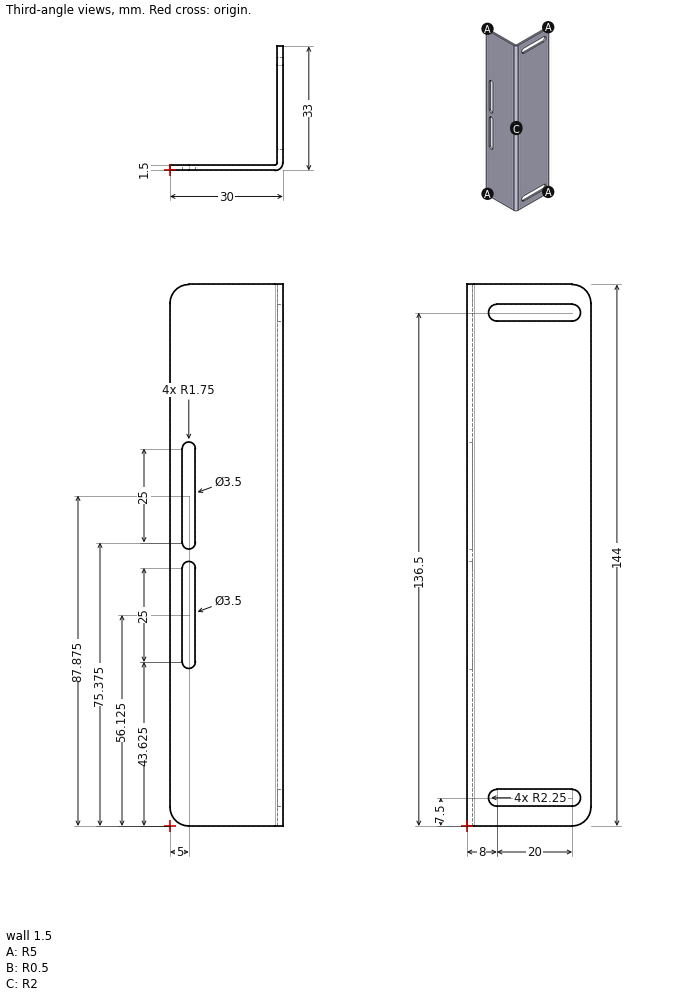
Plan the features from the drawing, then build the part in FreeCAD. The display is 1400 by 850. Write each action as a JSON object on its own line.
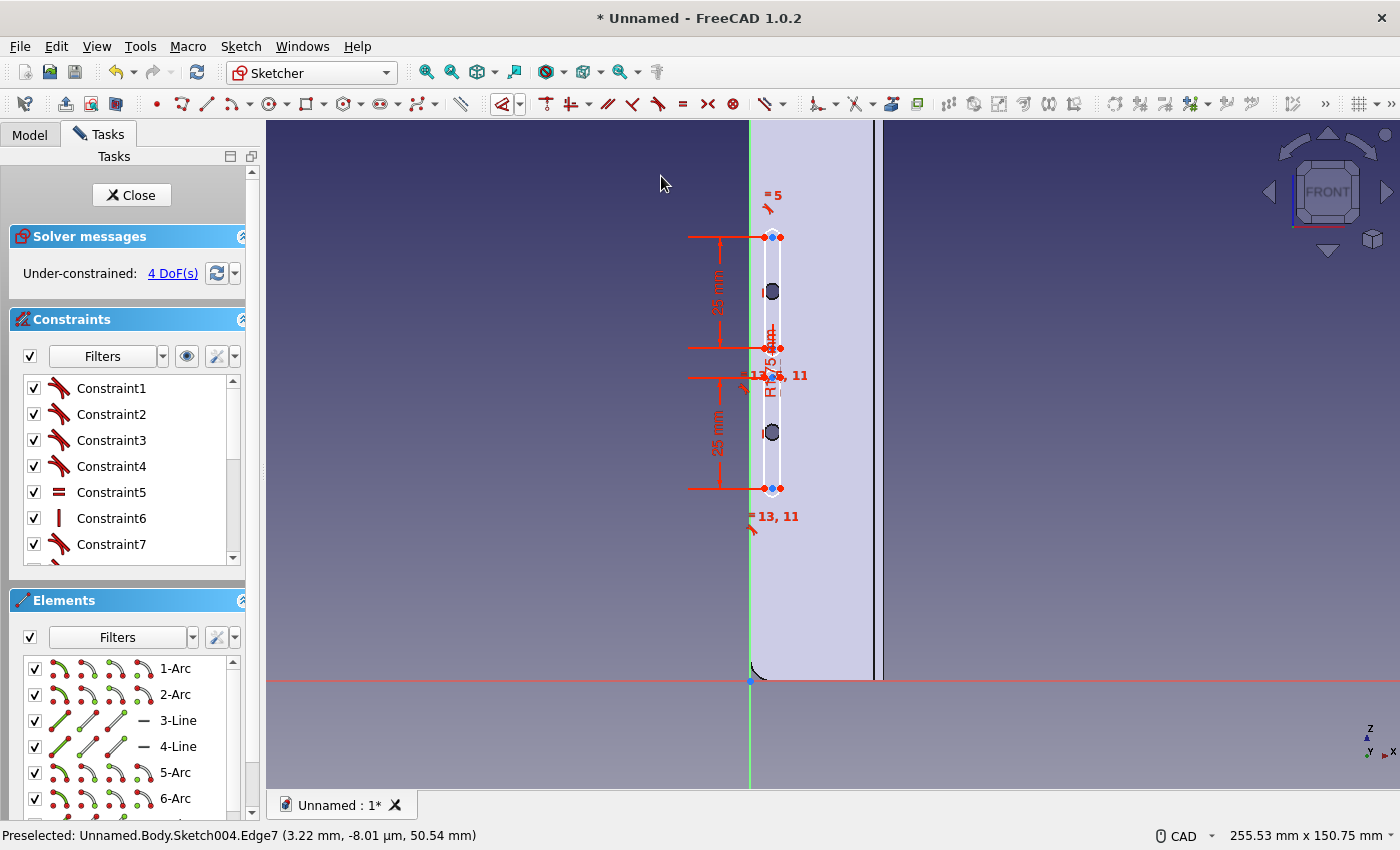
{"action": "scroll", "coordinate": [773, 348], "scroll_direction": "up", "scroll_amount": 3}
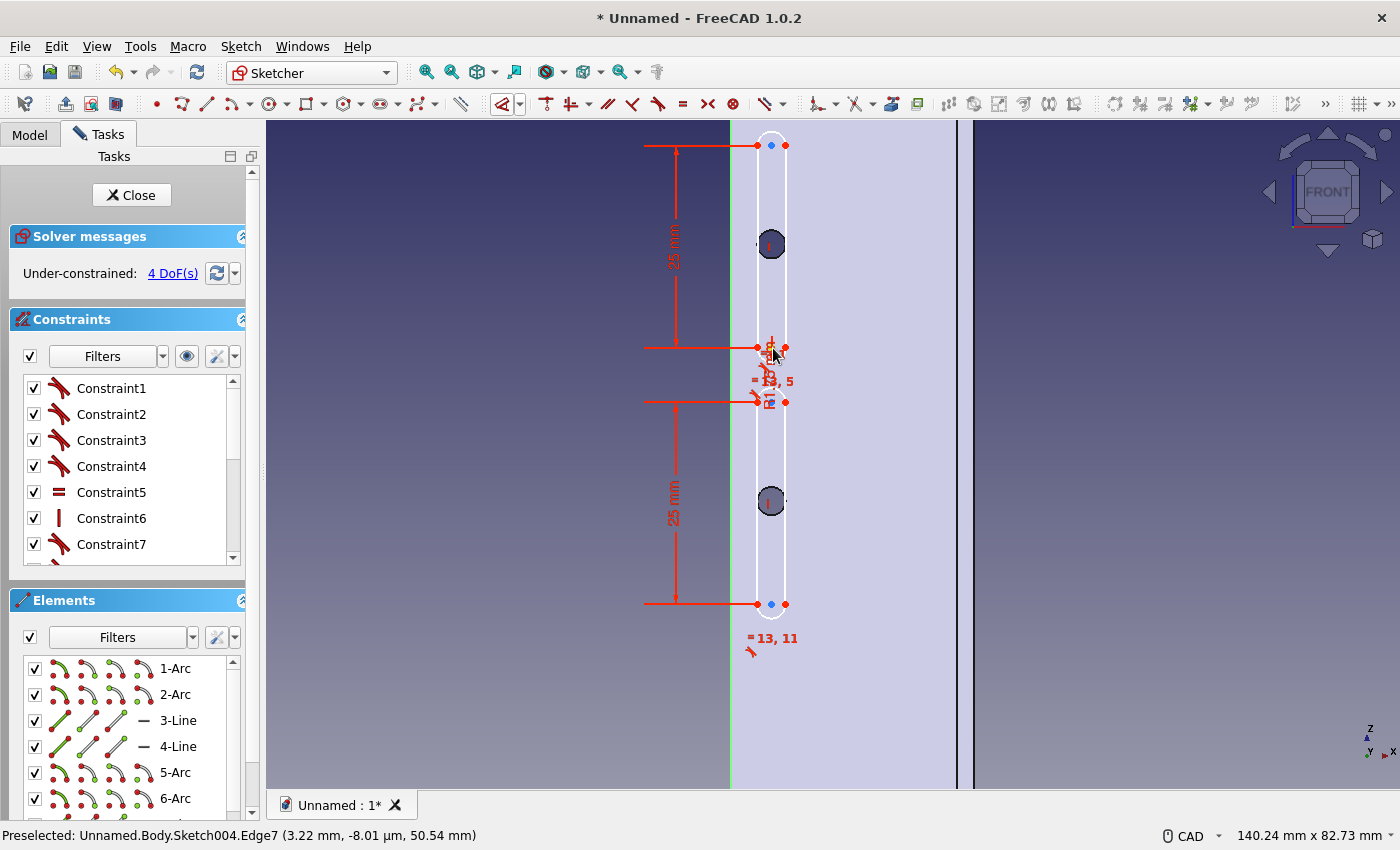
{"action": "scroll", "coordinate": [772, 348], "scroll_direction": "up", "scroll_amount": 4}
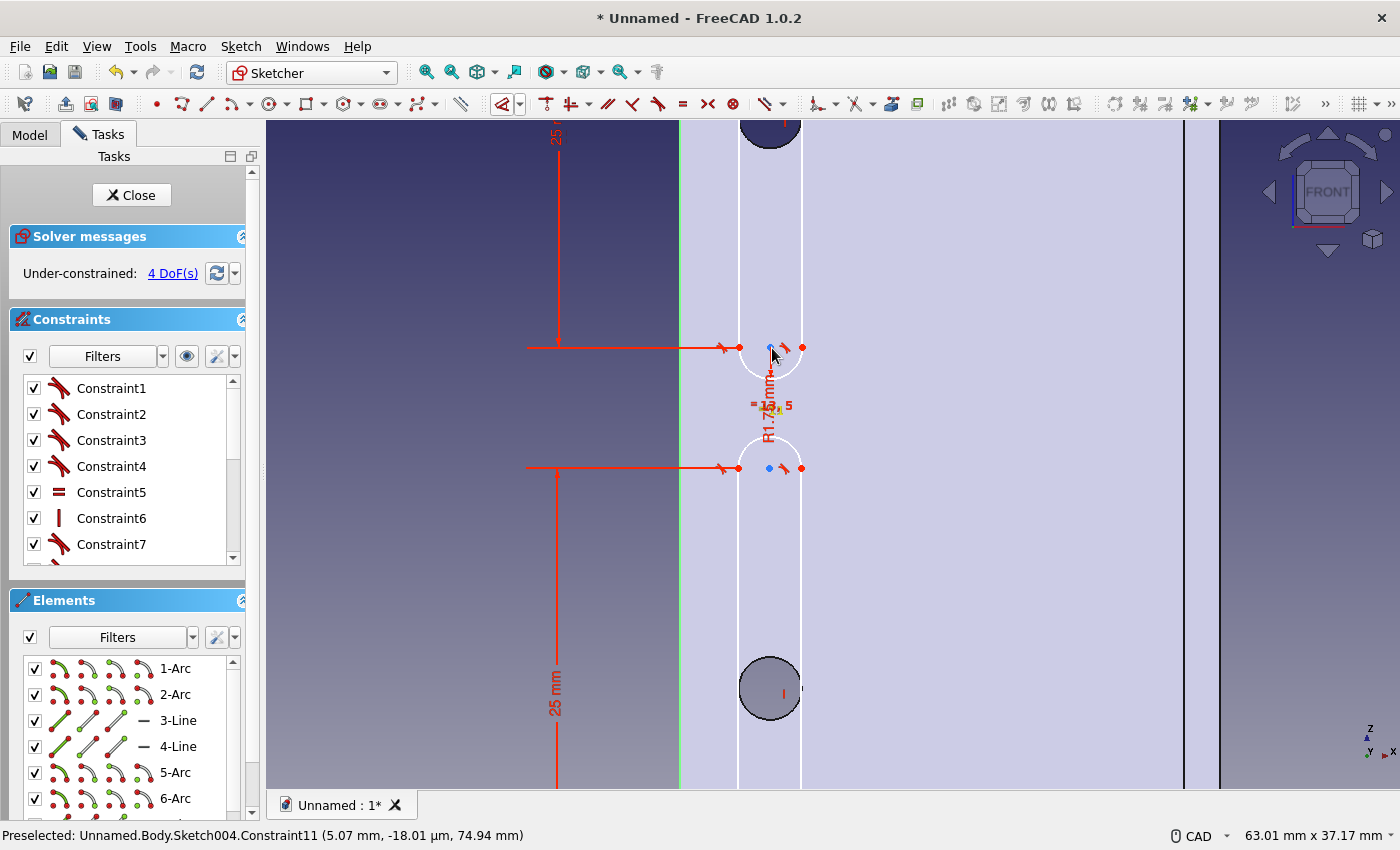
{"action": "left_click", "coordinate": [771, 348]}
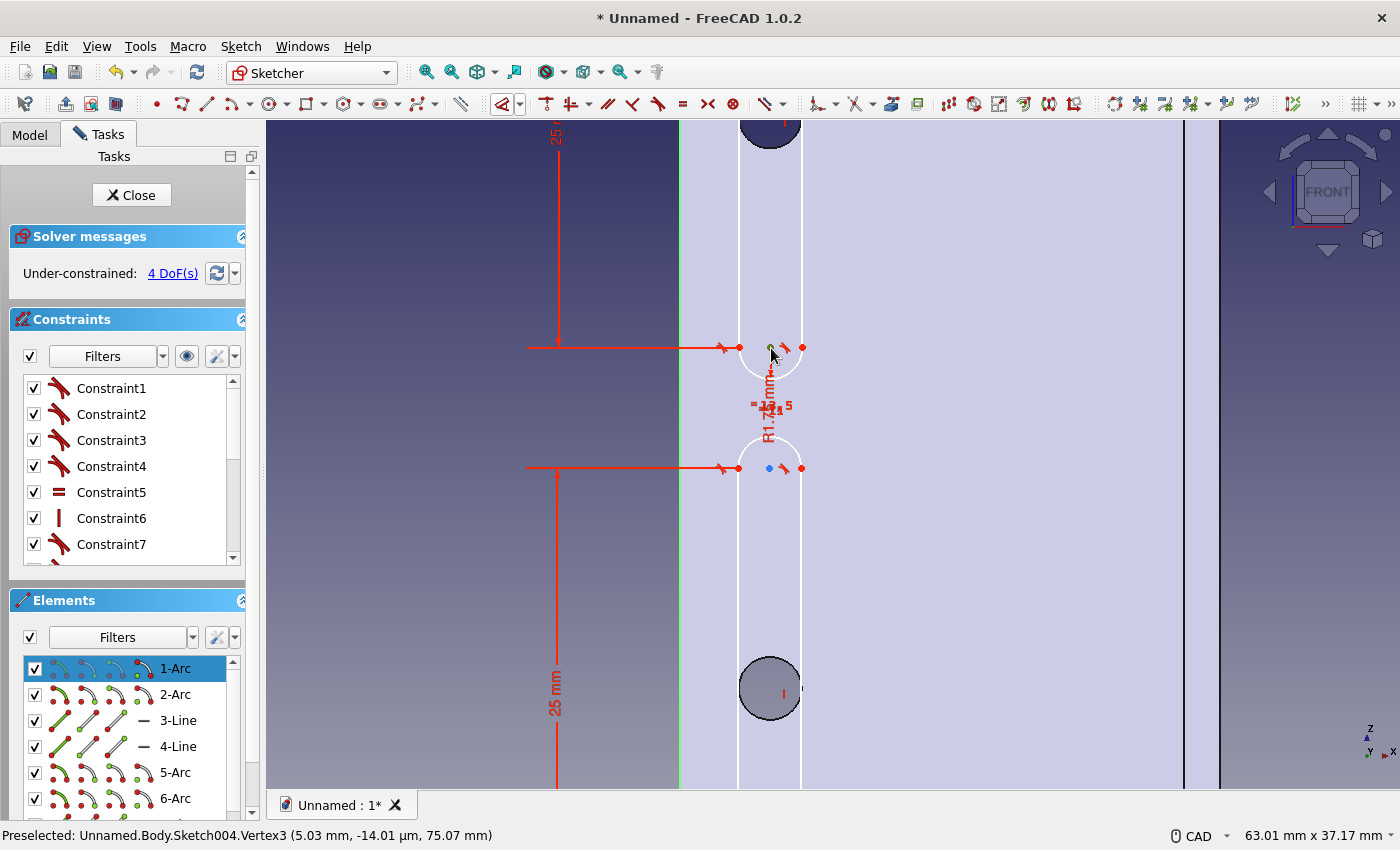
{"action": "key", "text": "l"}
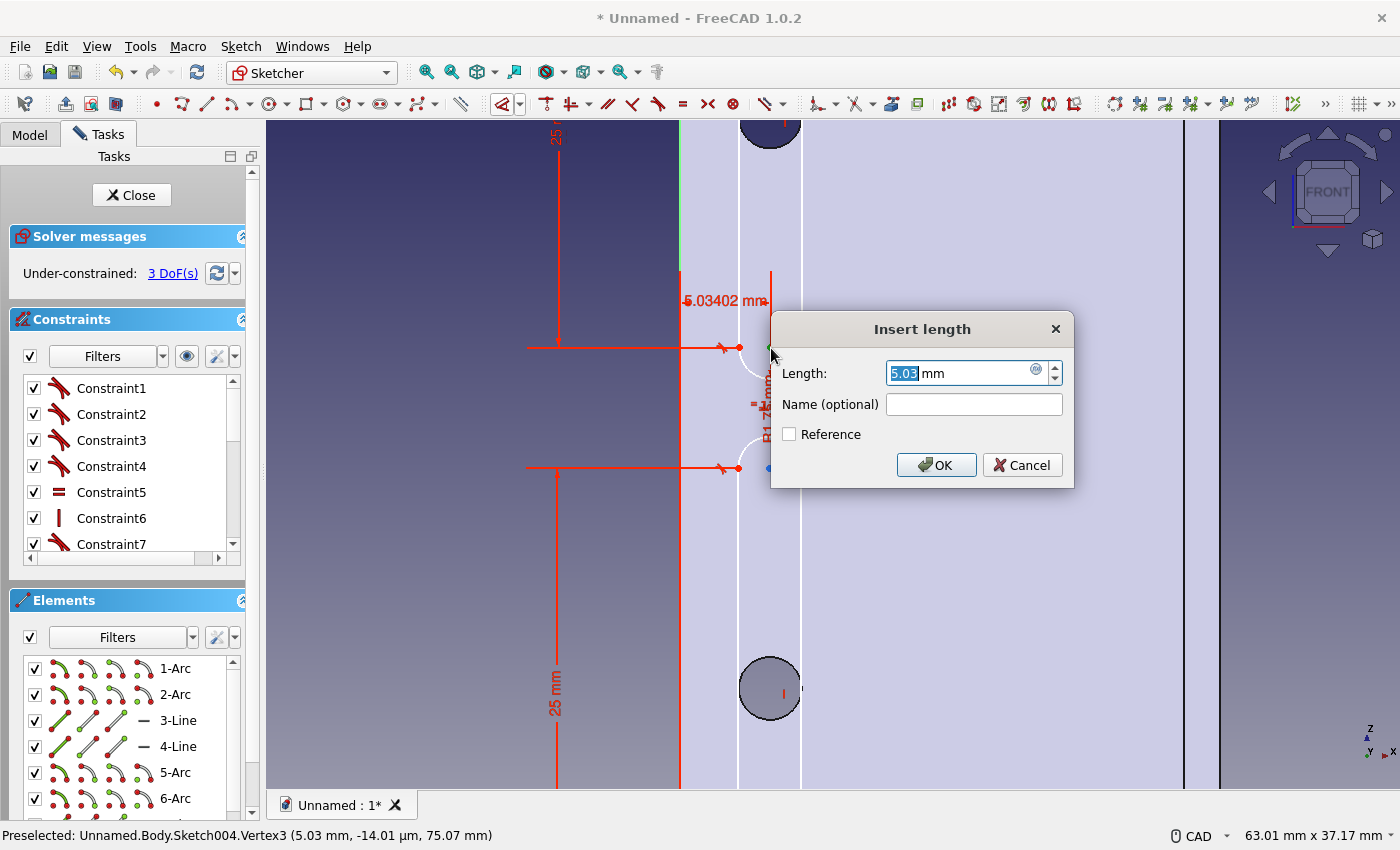
{"action": "type", "text": "5"}
{"action": "key", "text": "Return"}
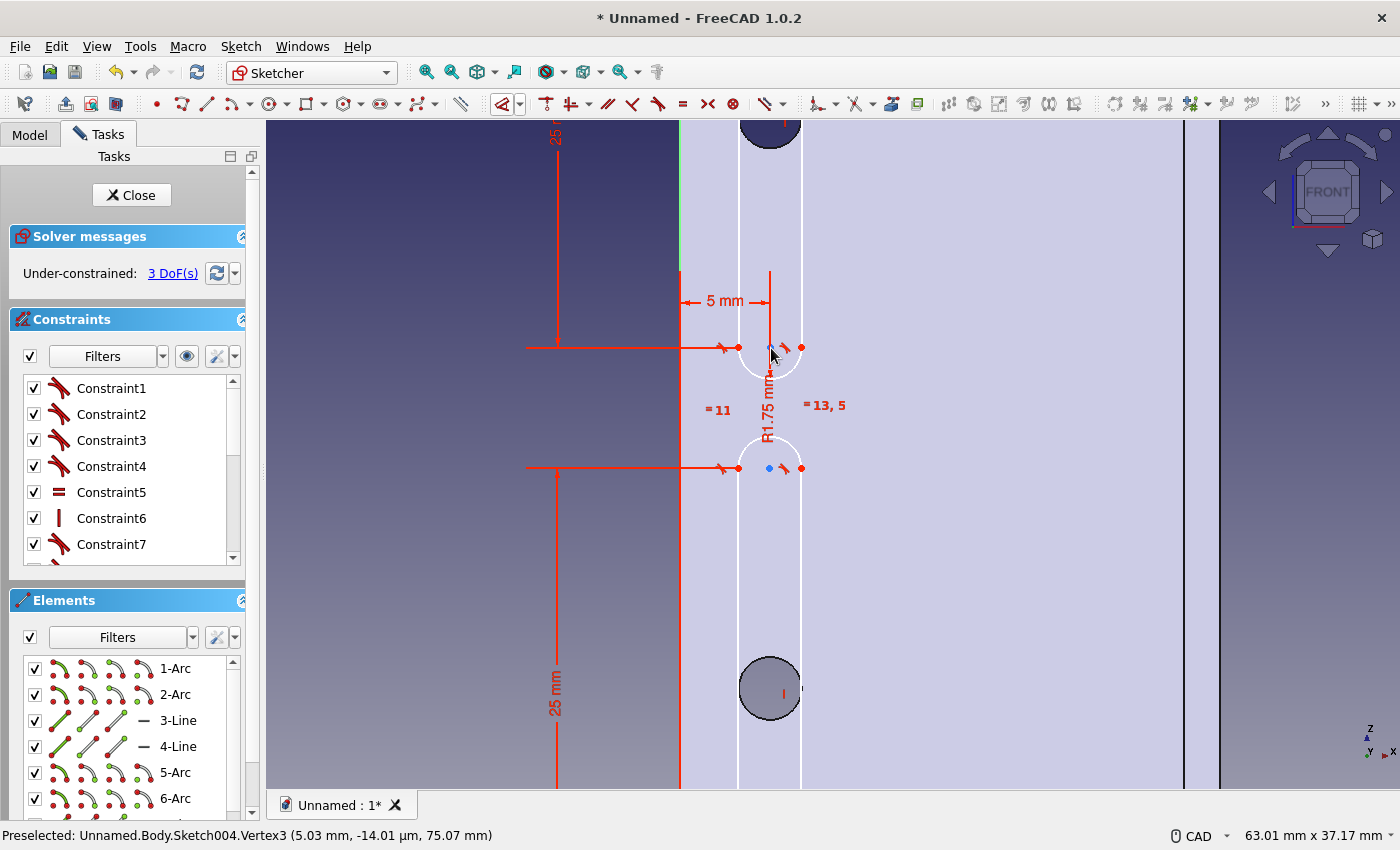
{"action": "scroll", "coordinate": [772, 348], "scroll_direction": "down", "scroll_amount": 7}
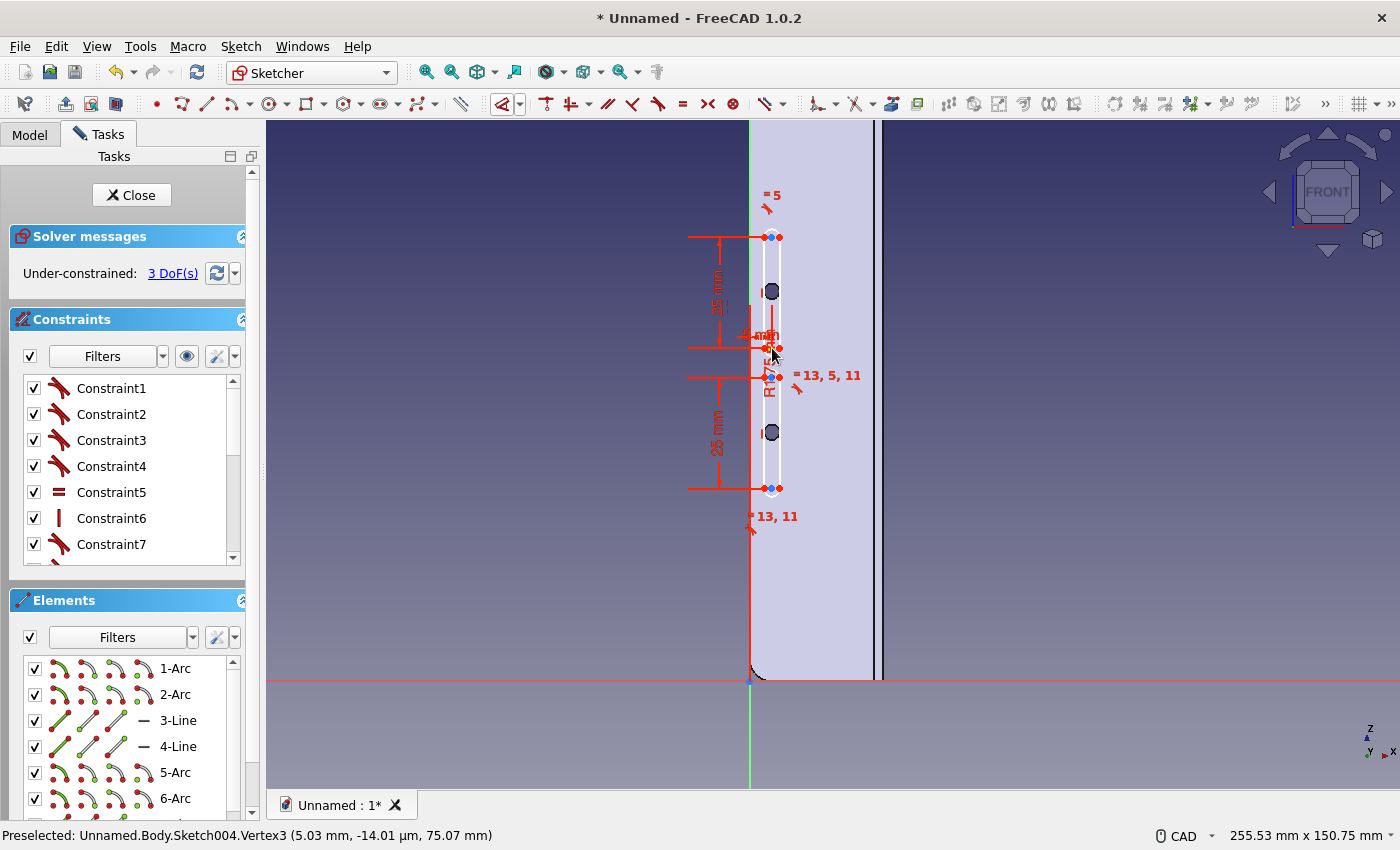
{"action": "scroll", "coordinate": [772, 489], "scroll_direction": "up", "scroll_amount": 3}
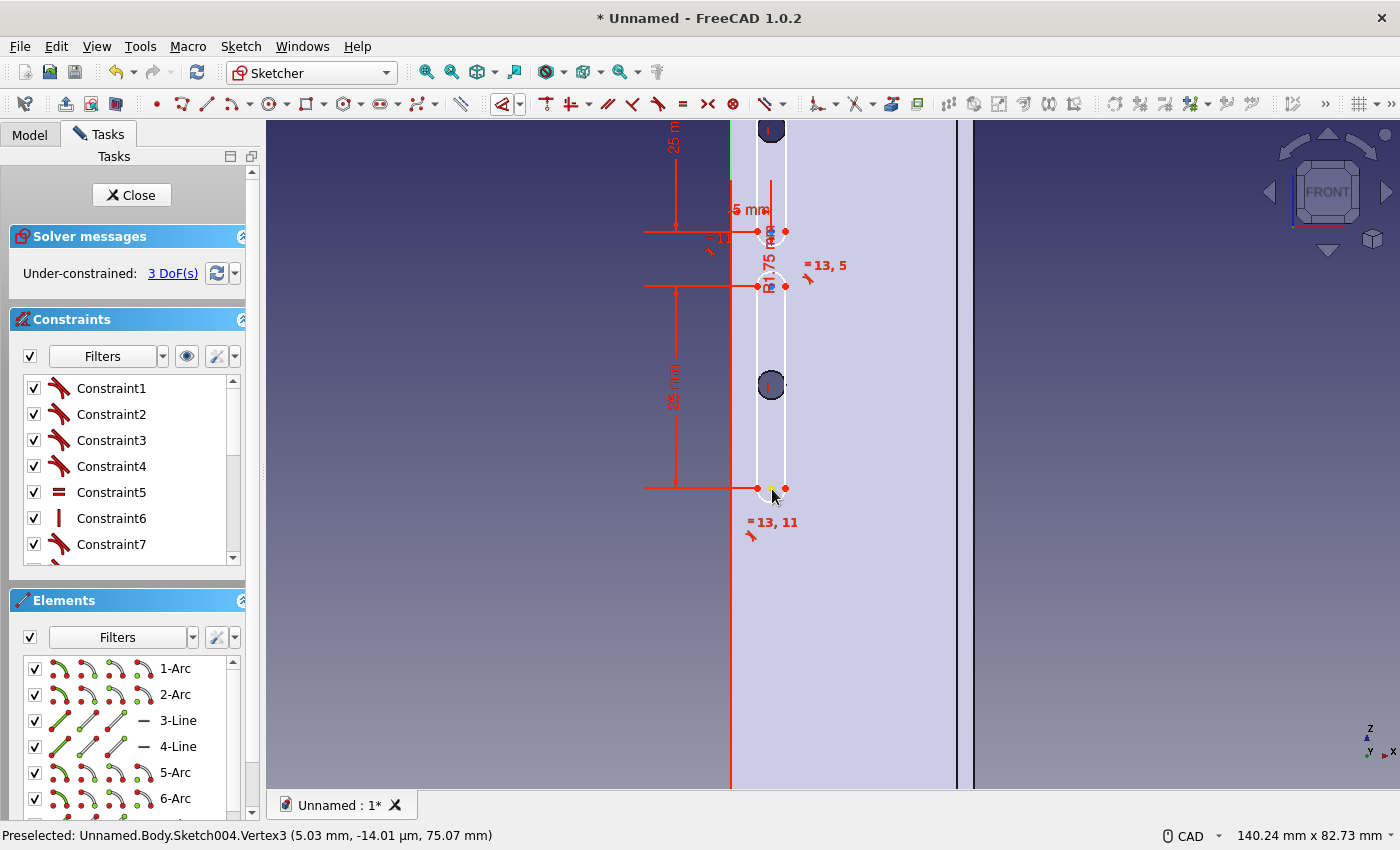
{"action": "left_click", "coordinate": [771, 488]}